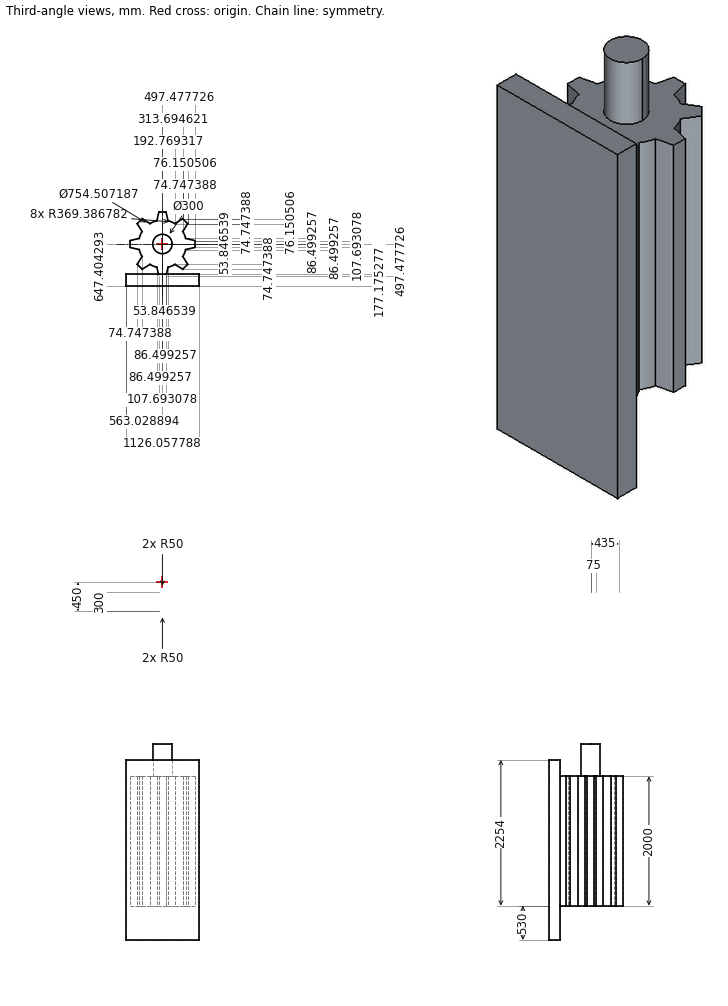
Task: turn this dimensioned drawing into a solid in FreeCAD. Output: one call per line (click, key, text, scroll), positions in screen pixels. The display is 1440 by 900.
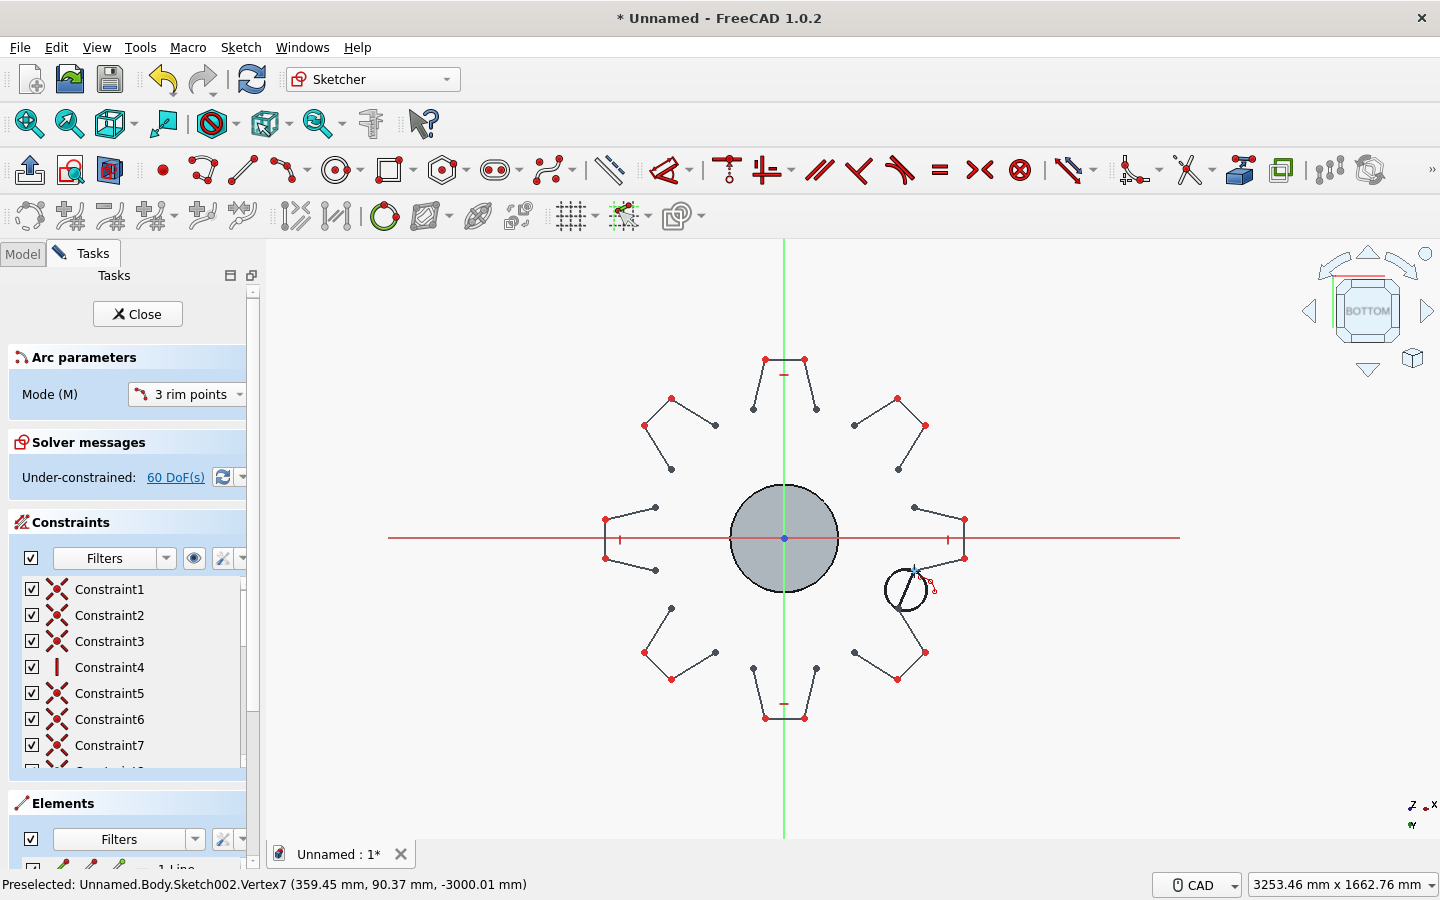
scroll(907, 589, up, 12)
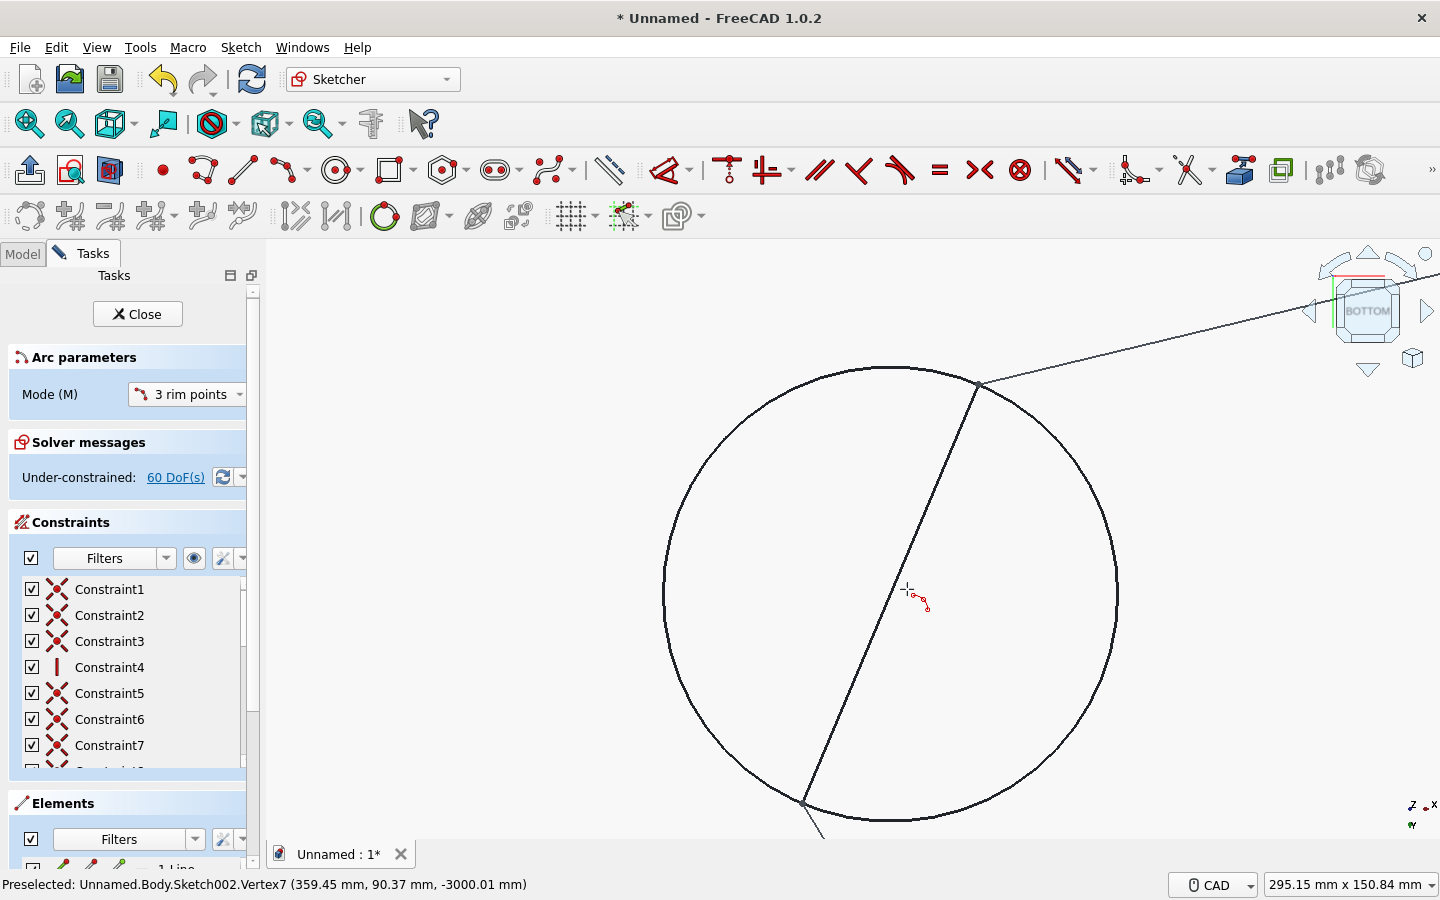
click(906, 588)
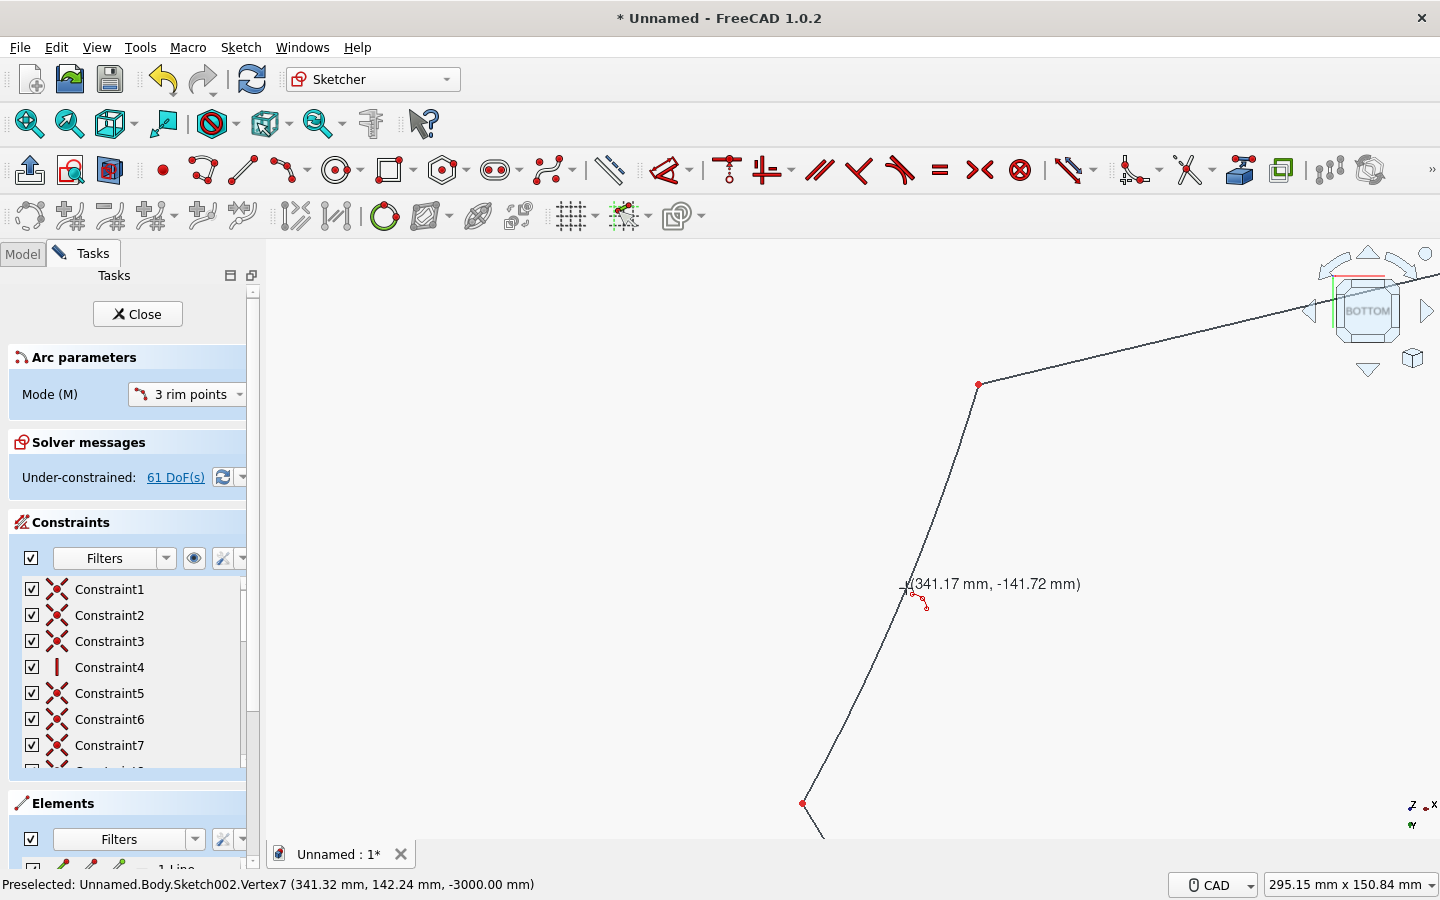
scroll(908, 590, down, 12)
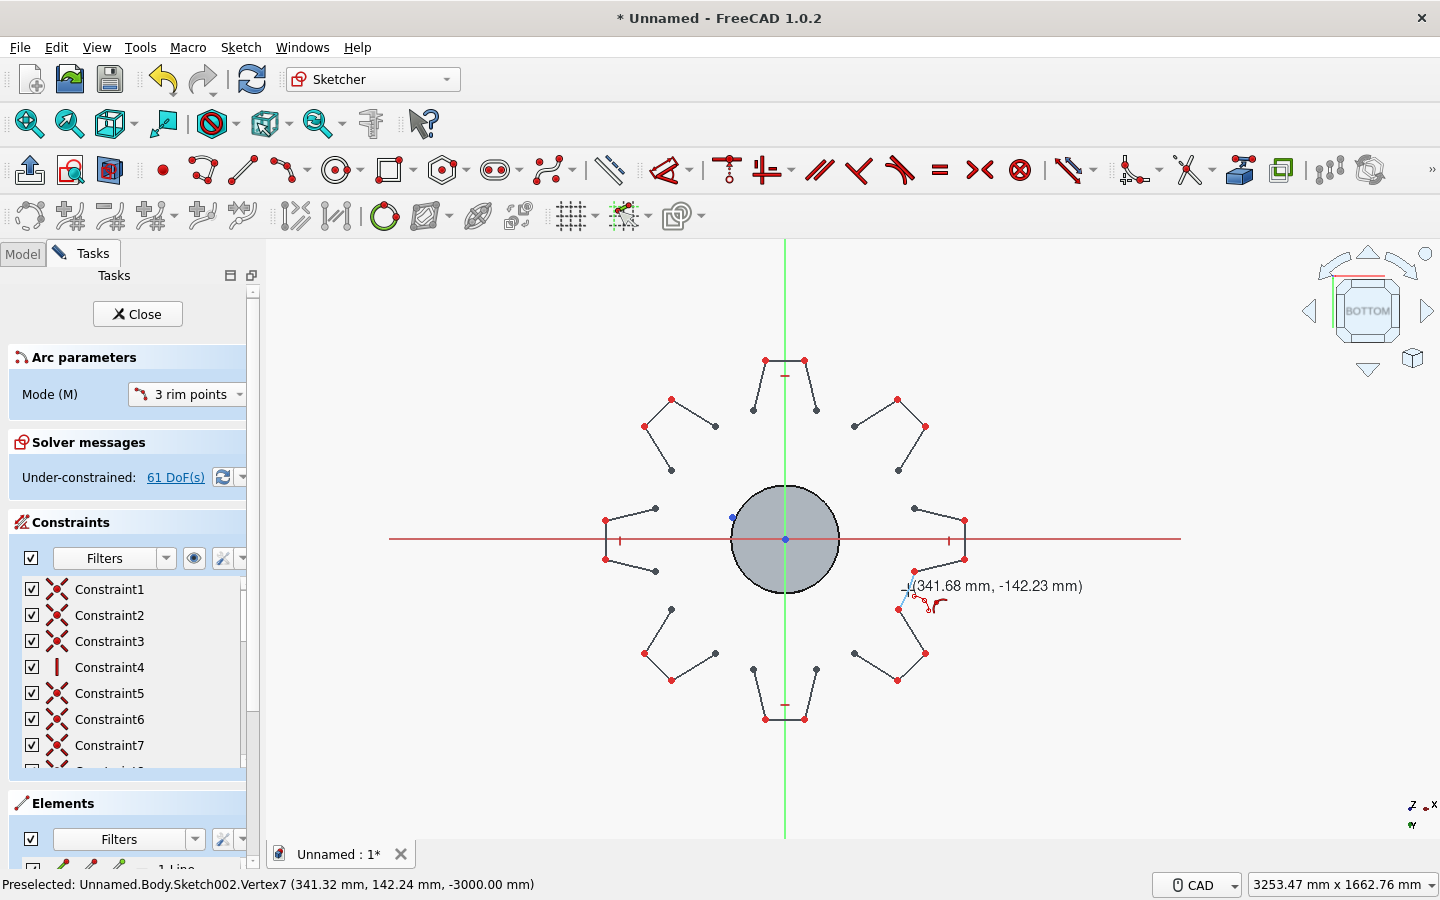
click(915, 509)
click(899, 471)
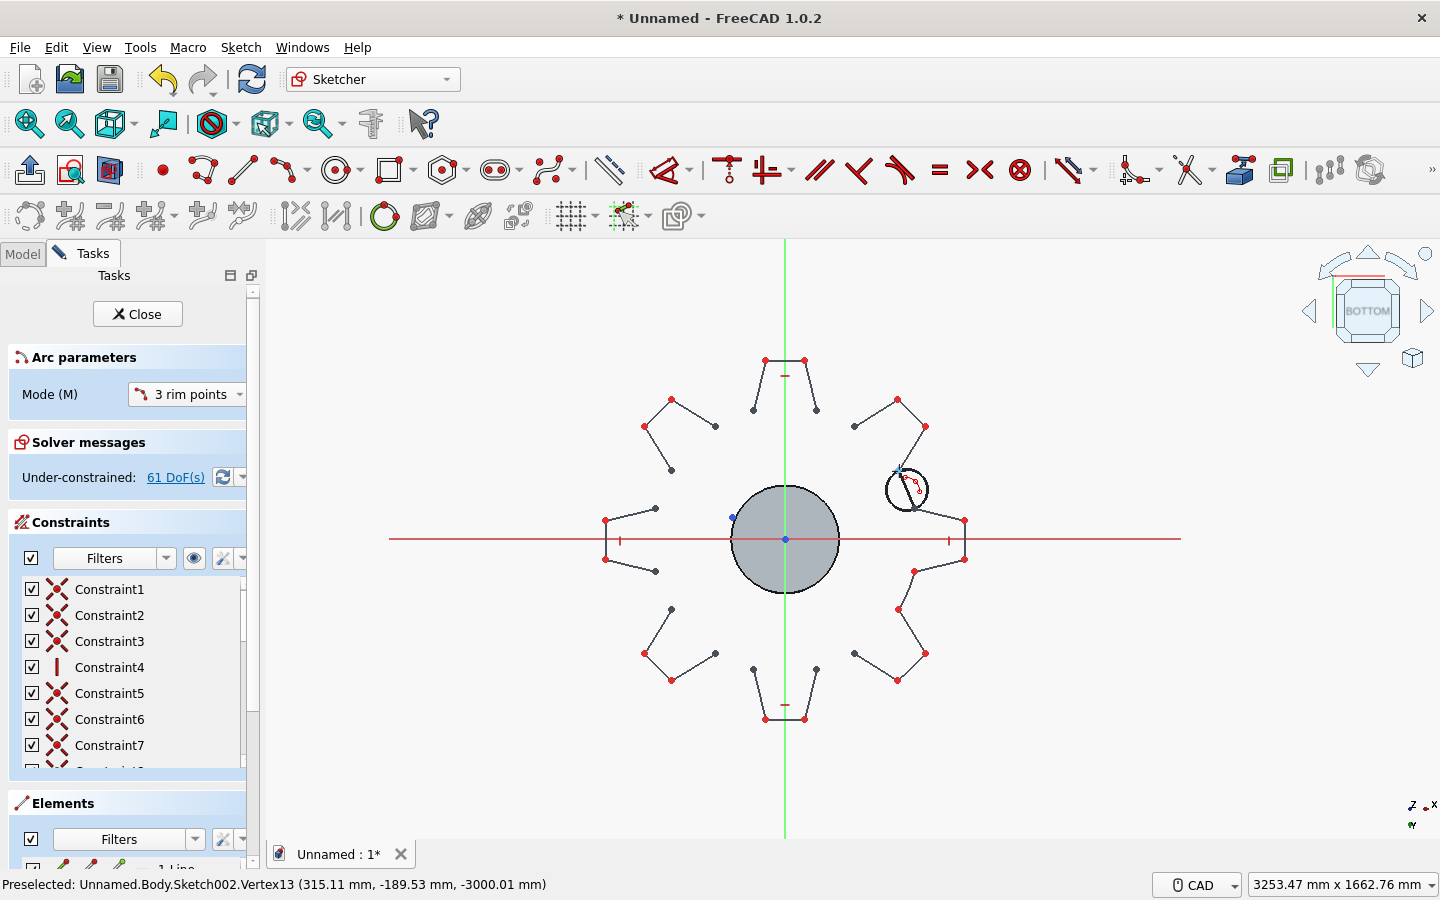
scroll(908, 488, up, 12)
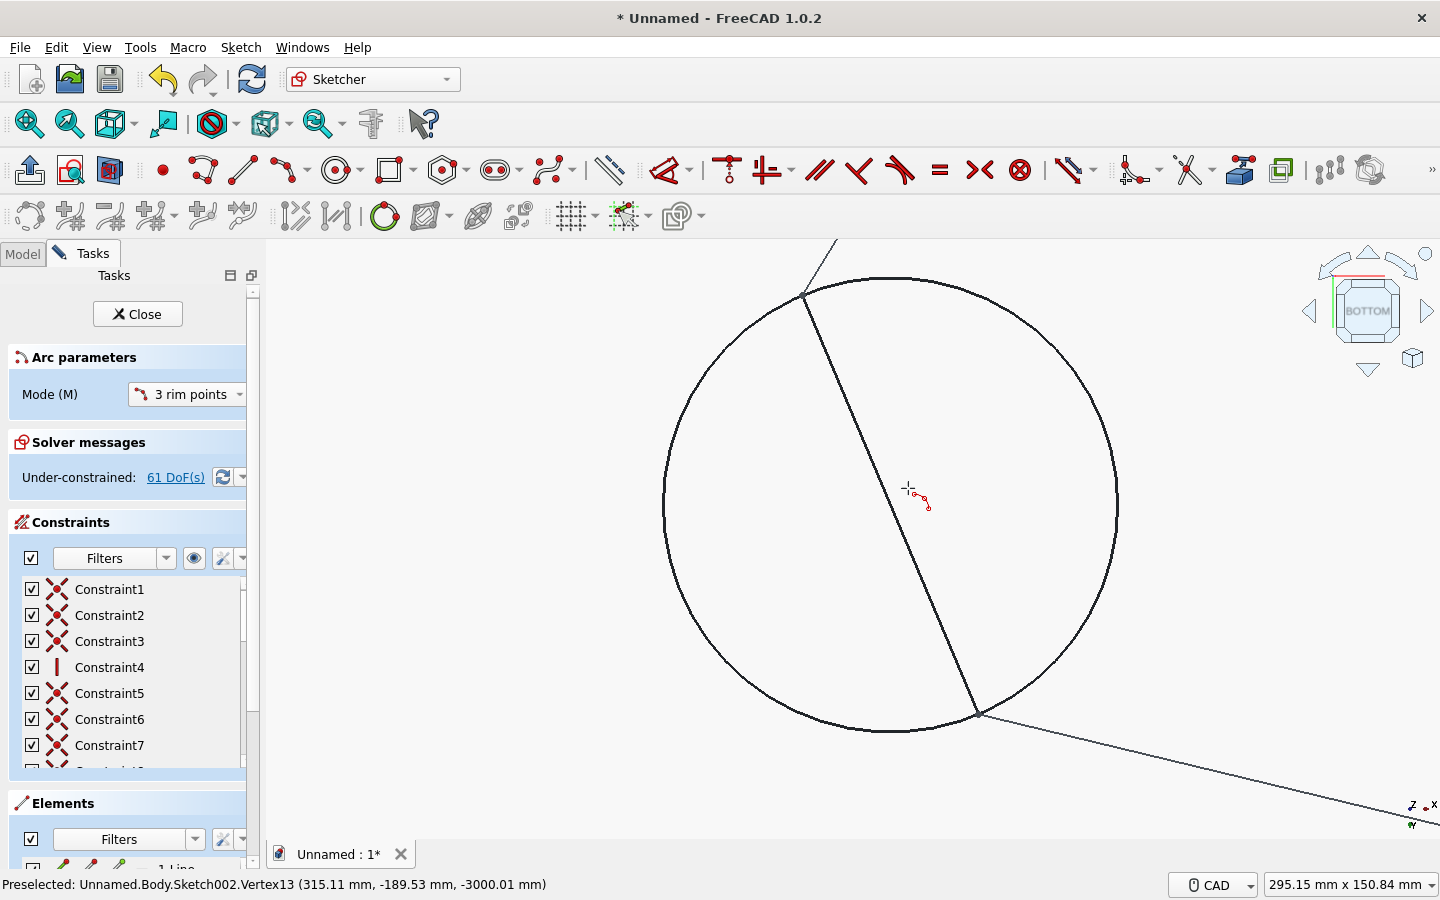
click(906, 487)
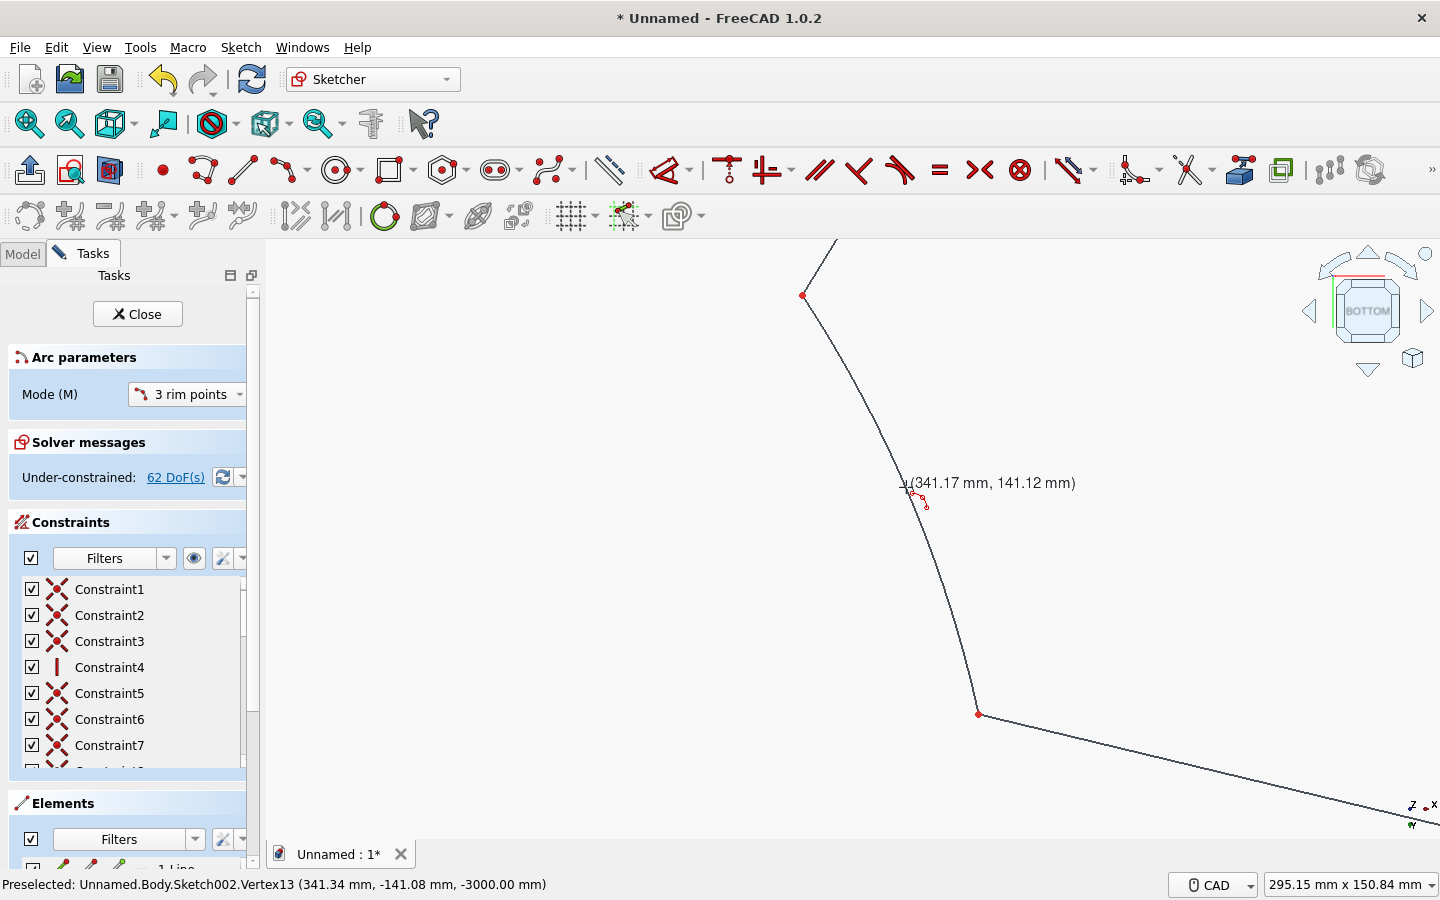
scroll(908, 488, down, 12)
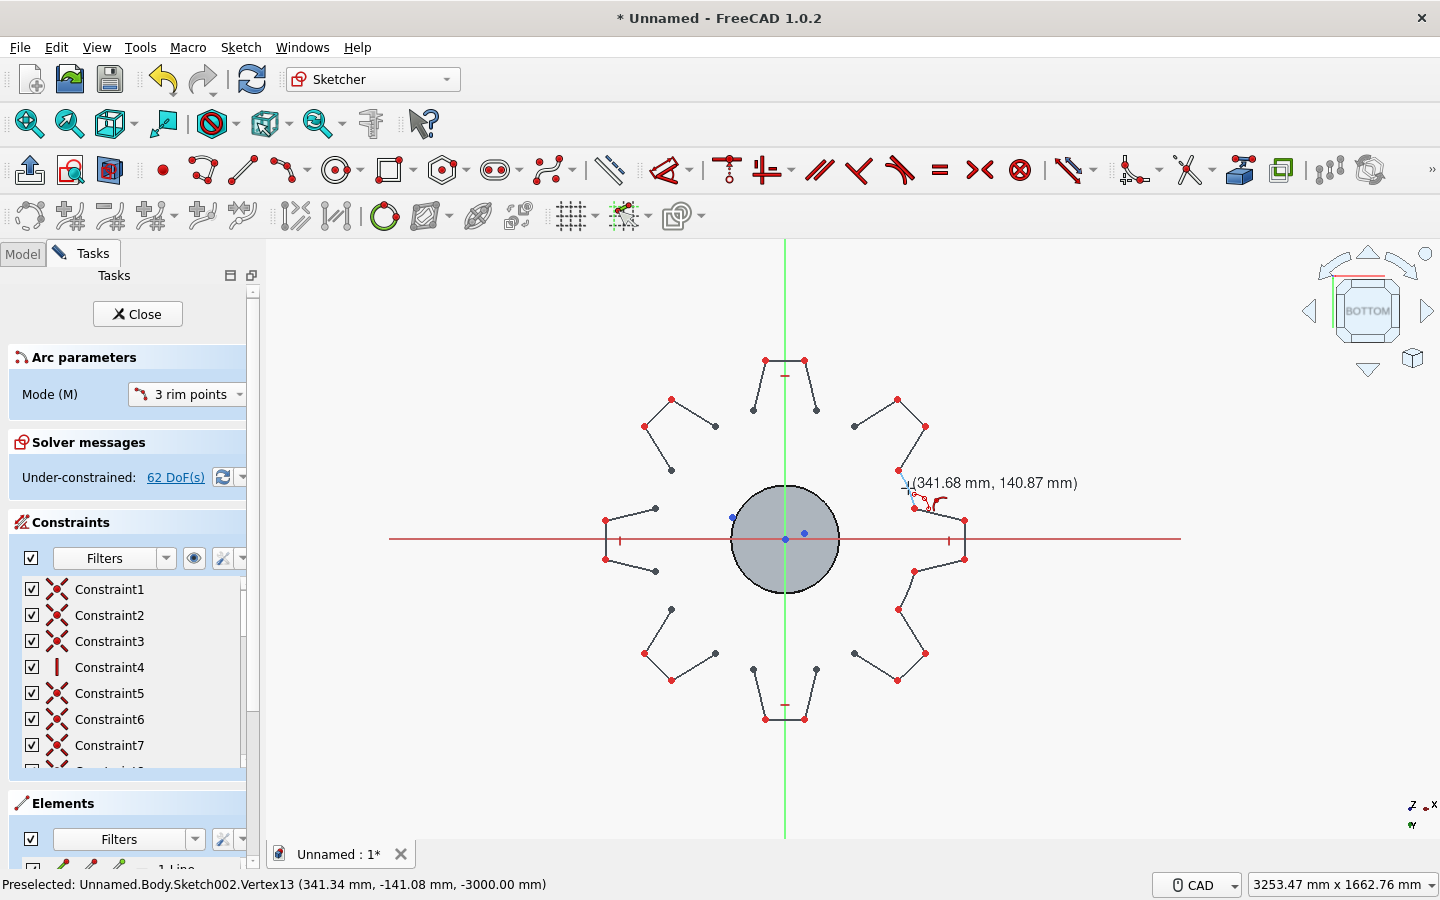
click(855, 427)
click(817, 411)